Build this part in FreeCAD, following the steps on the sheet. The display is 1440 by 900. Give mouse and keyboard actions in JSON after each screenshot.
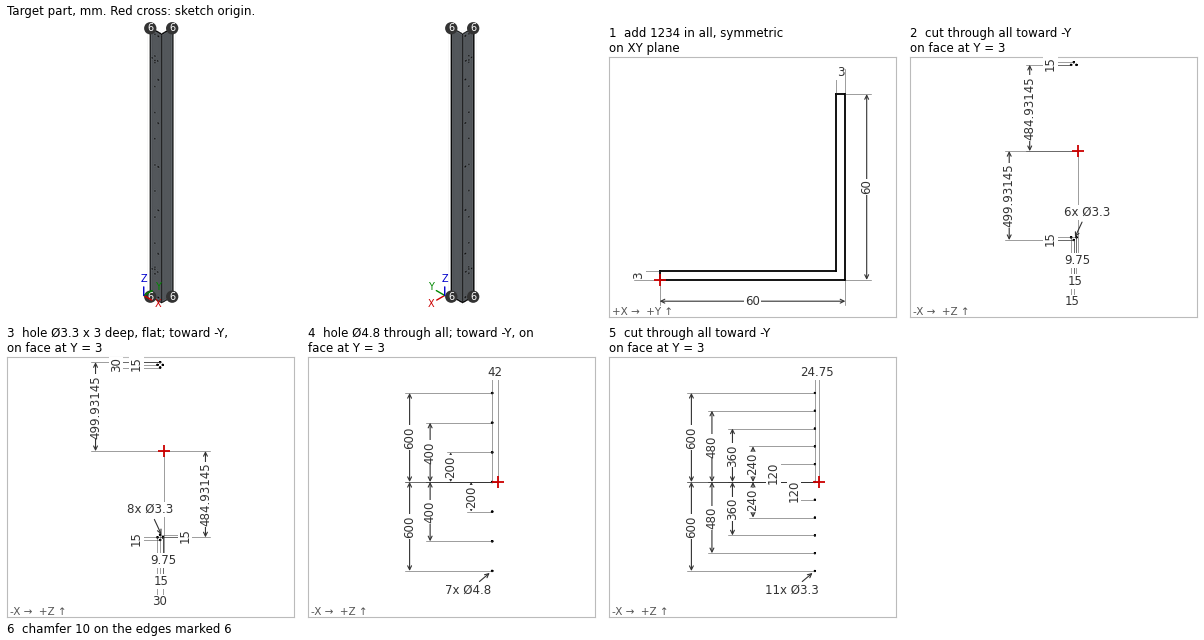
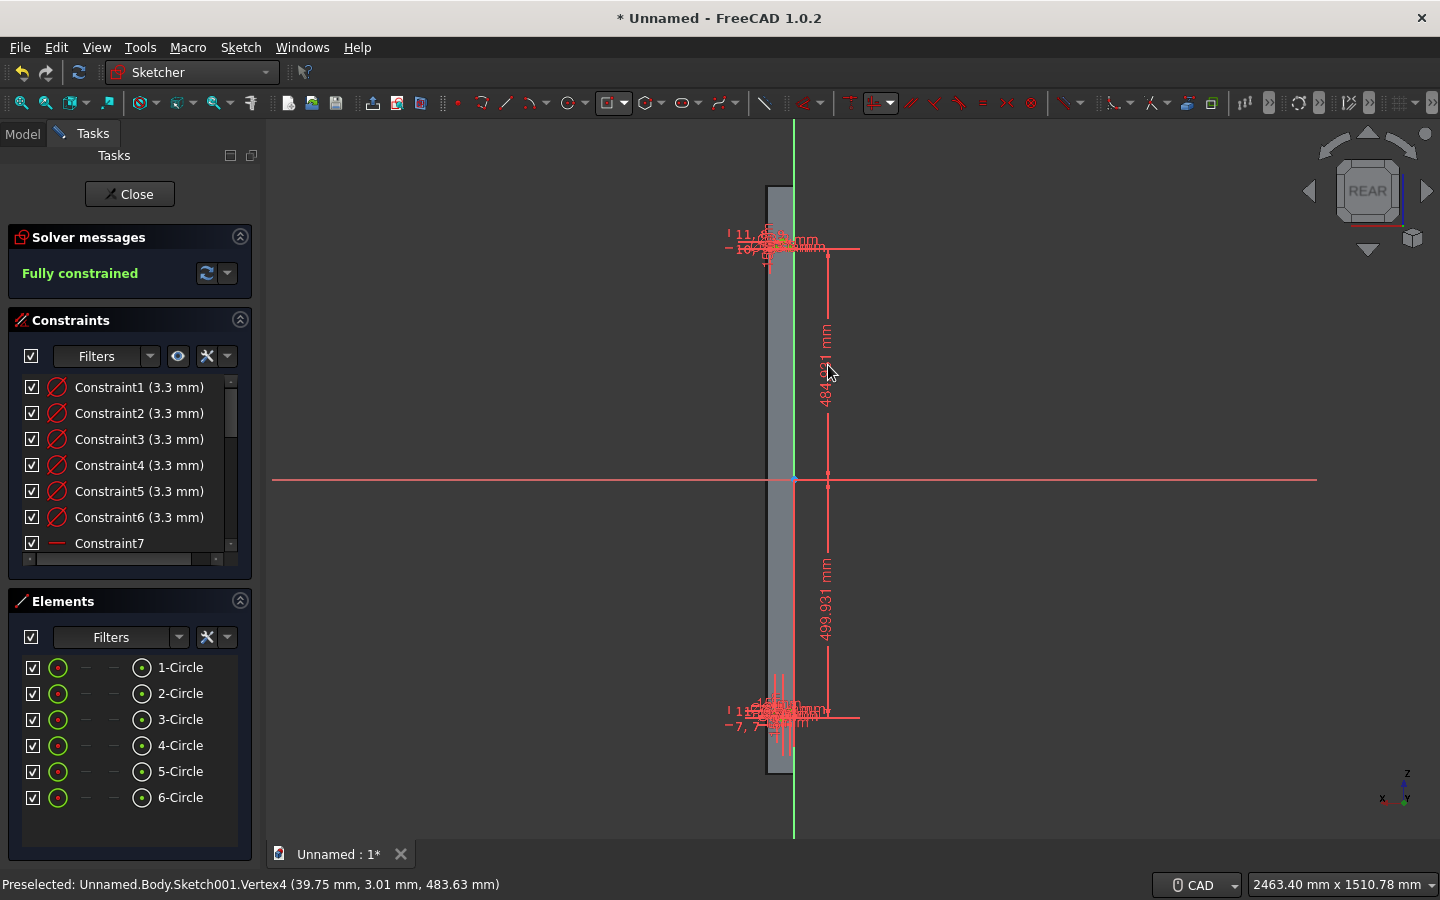
{"action": "left_click", "coordinate": [130, 194]}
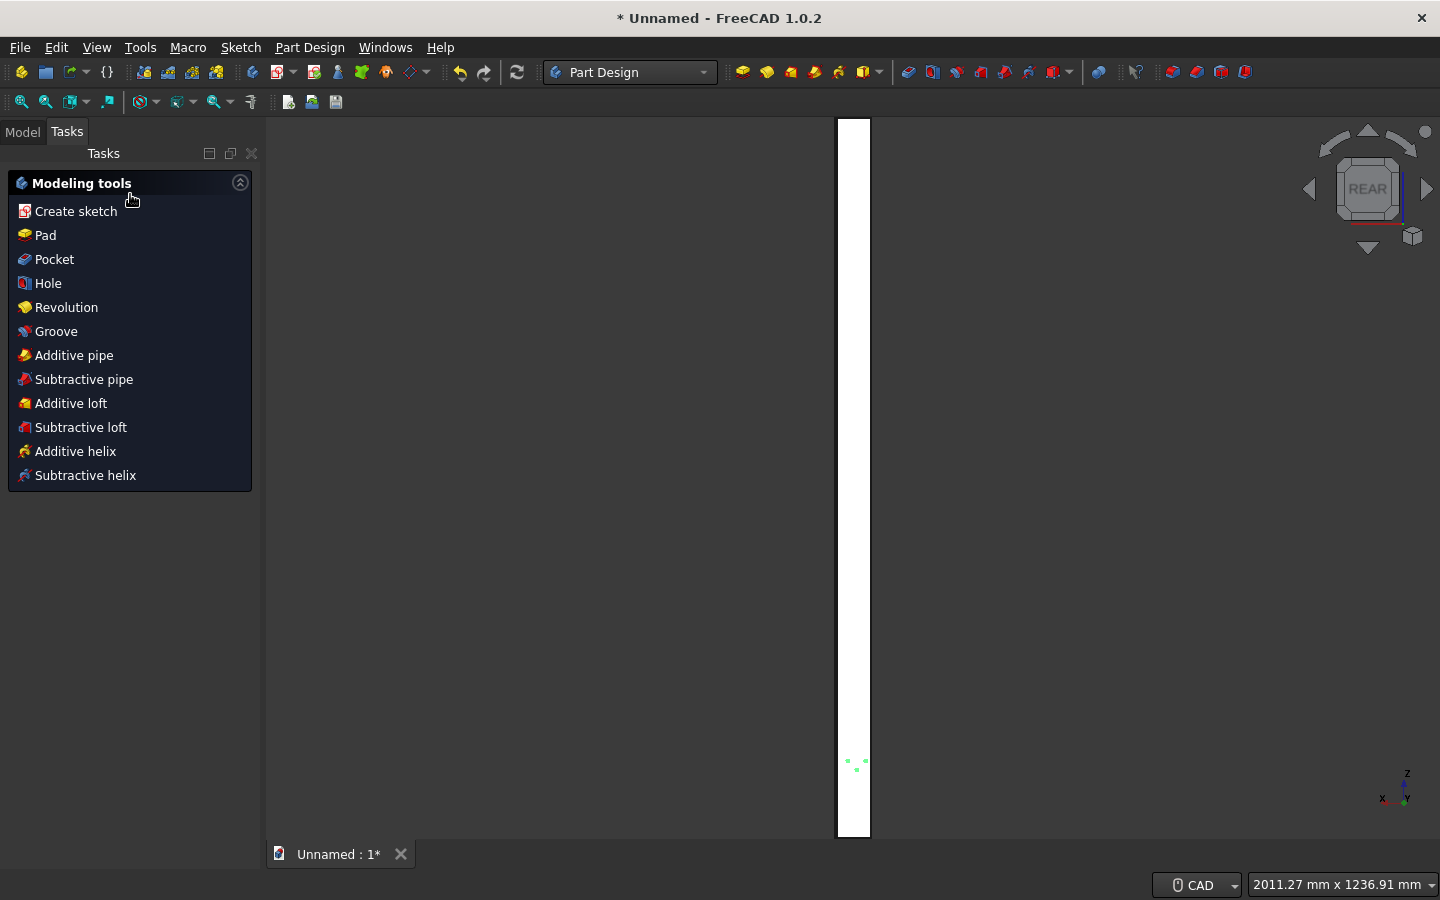
{"action": "left_click", "coordinate": [910, 72]}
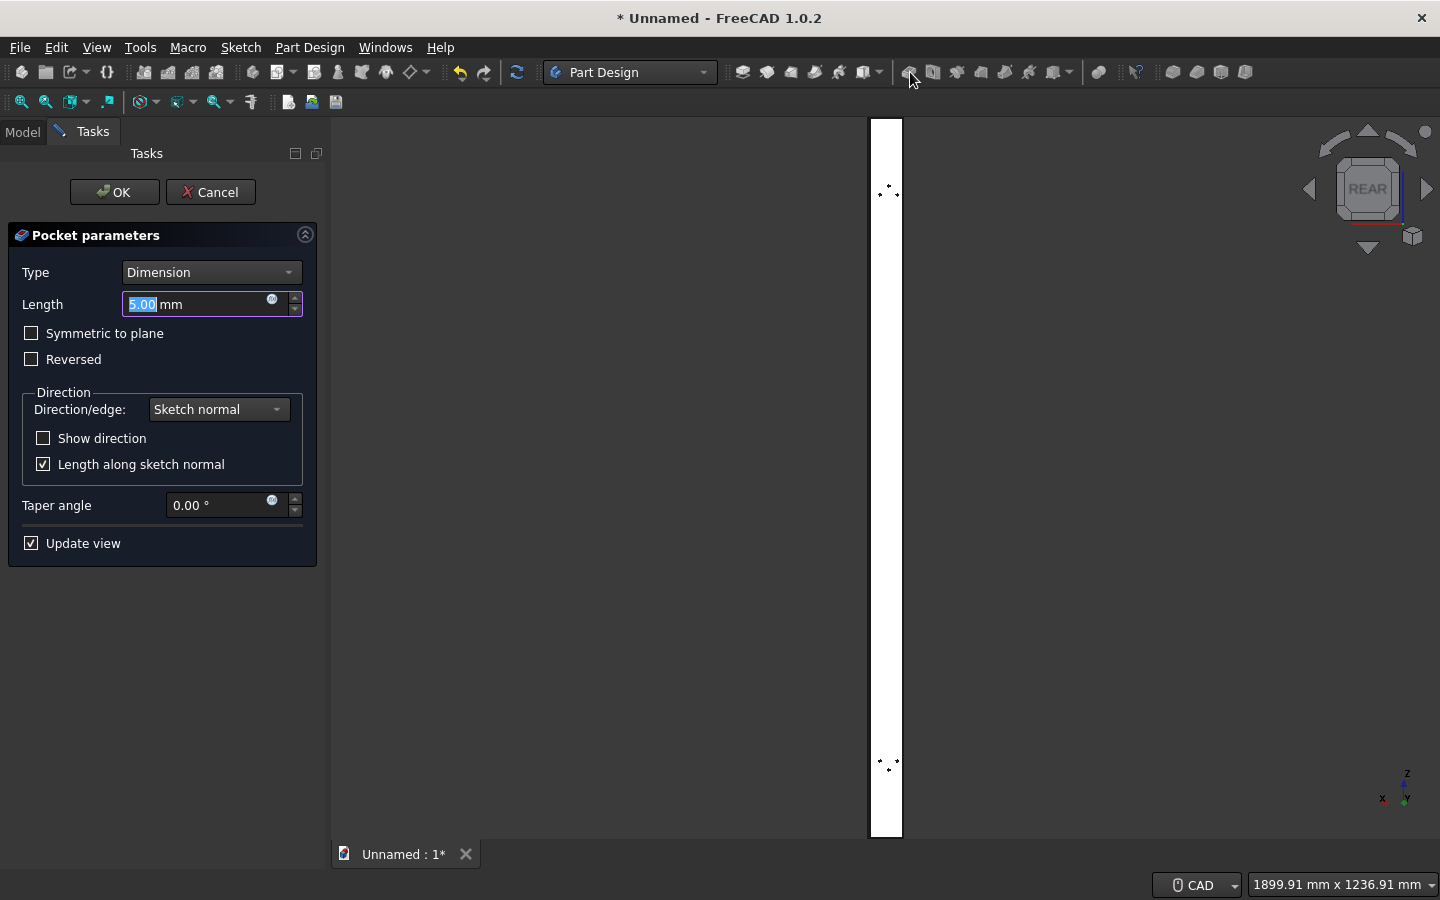
{"action": "left_click", "coordinate": [212, 272]}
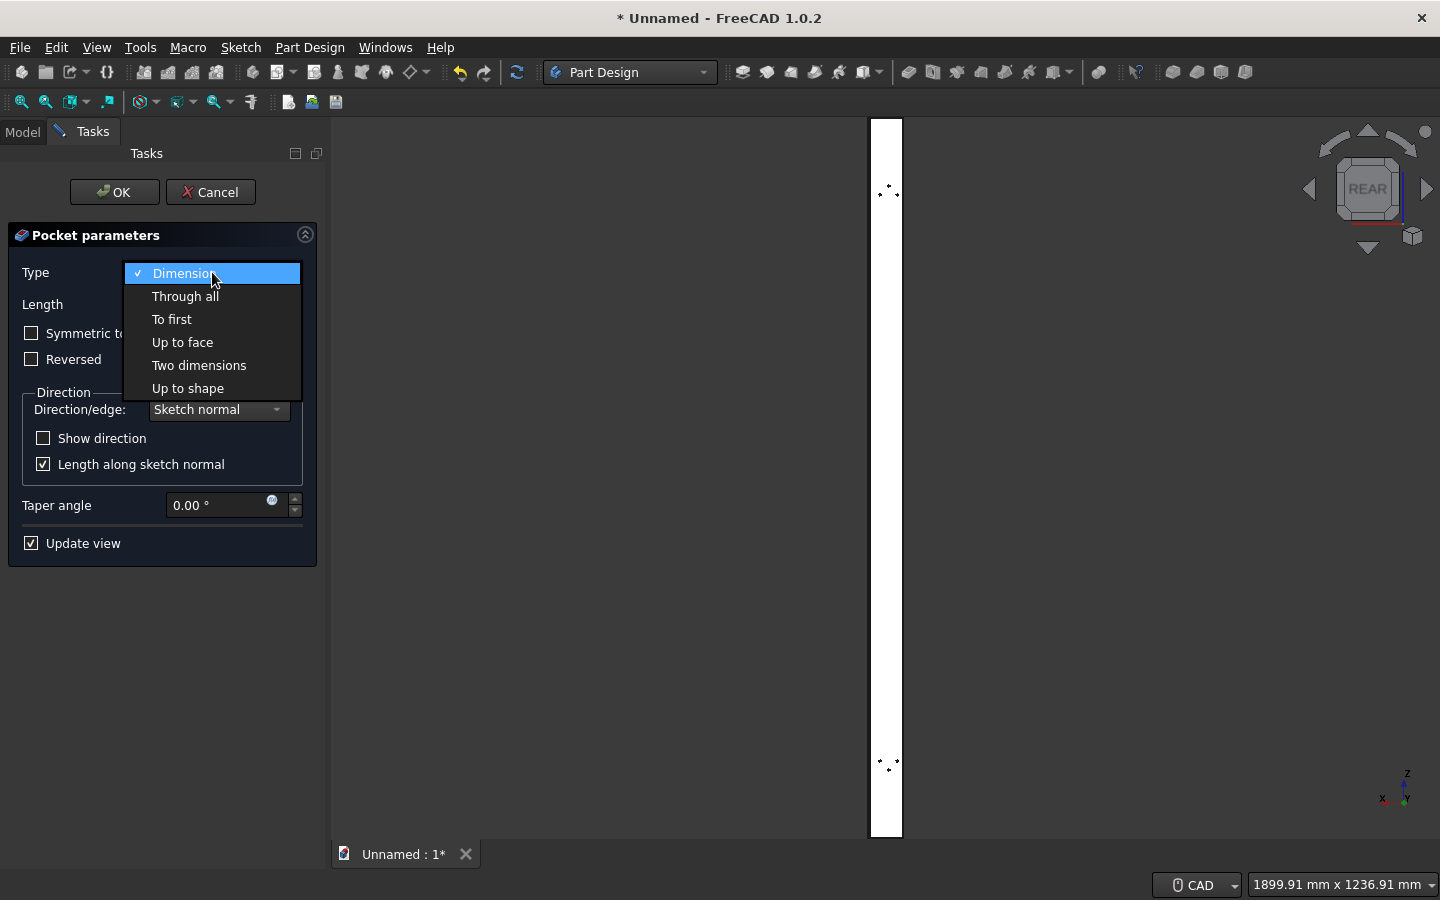
{"action": "left_click", "coordinate": [212, 296]}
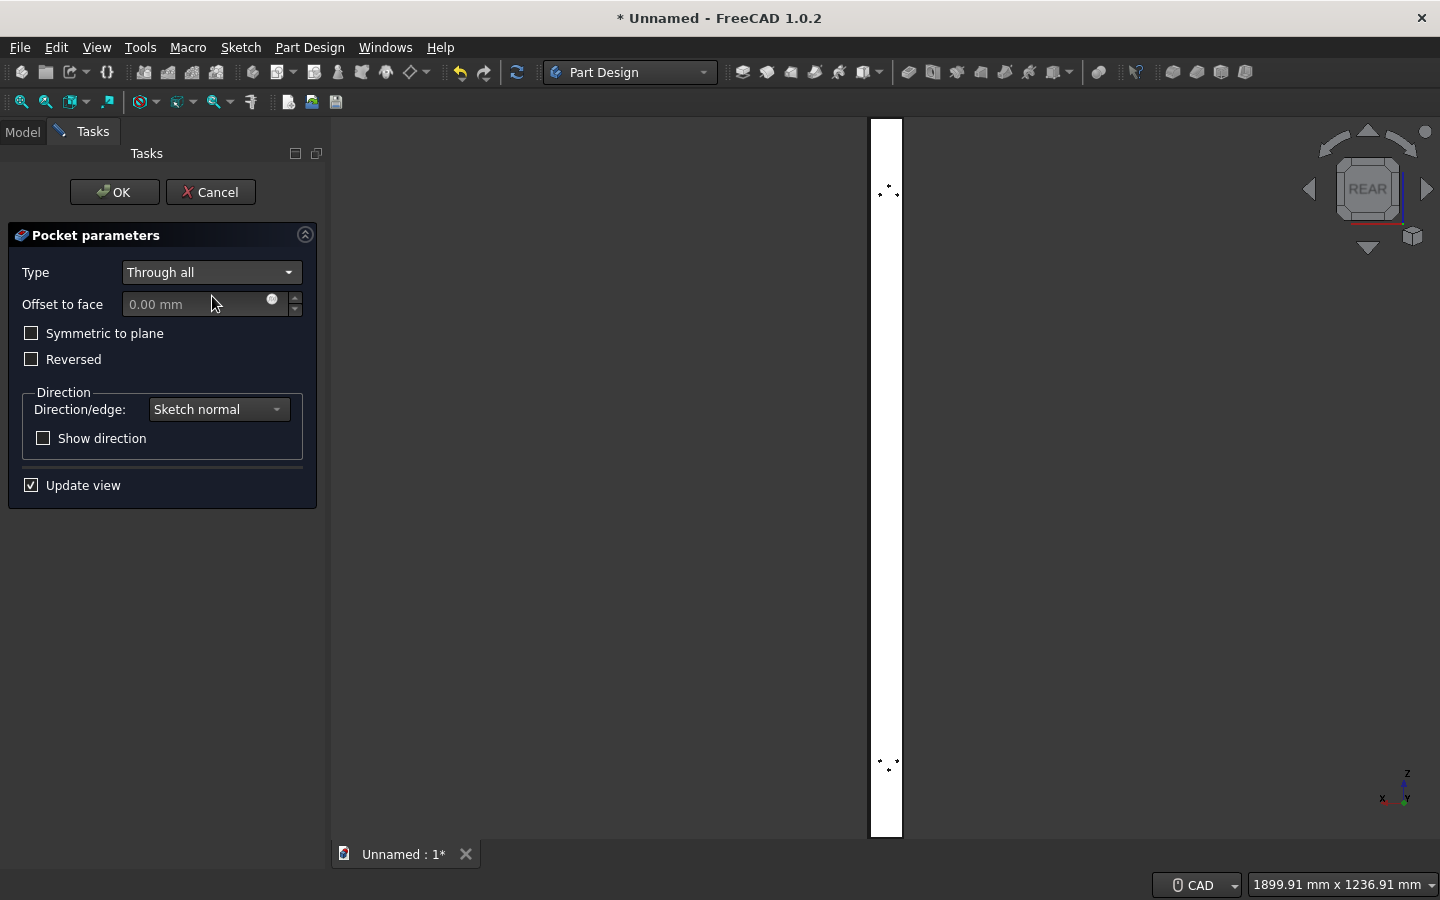
{"action": "left_click", "coordinate": [115, 192]}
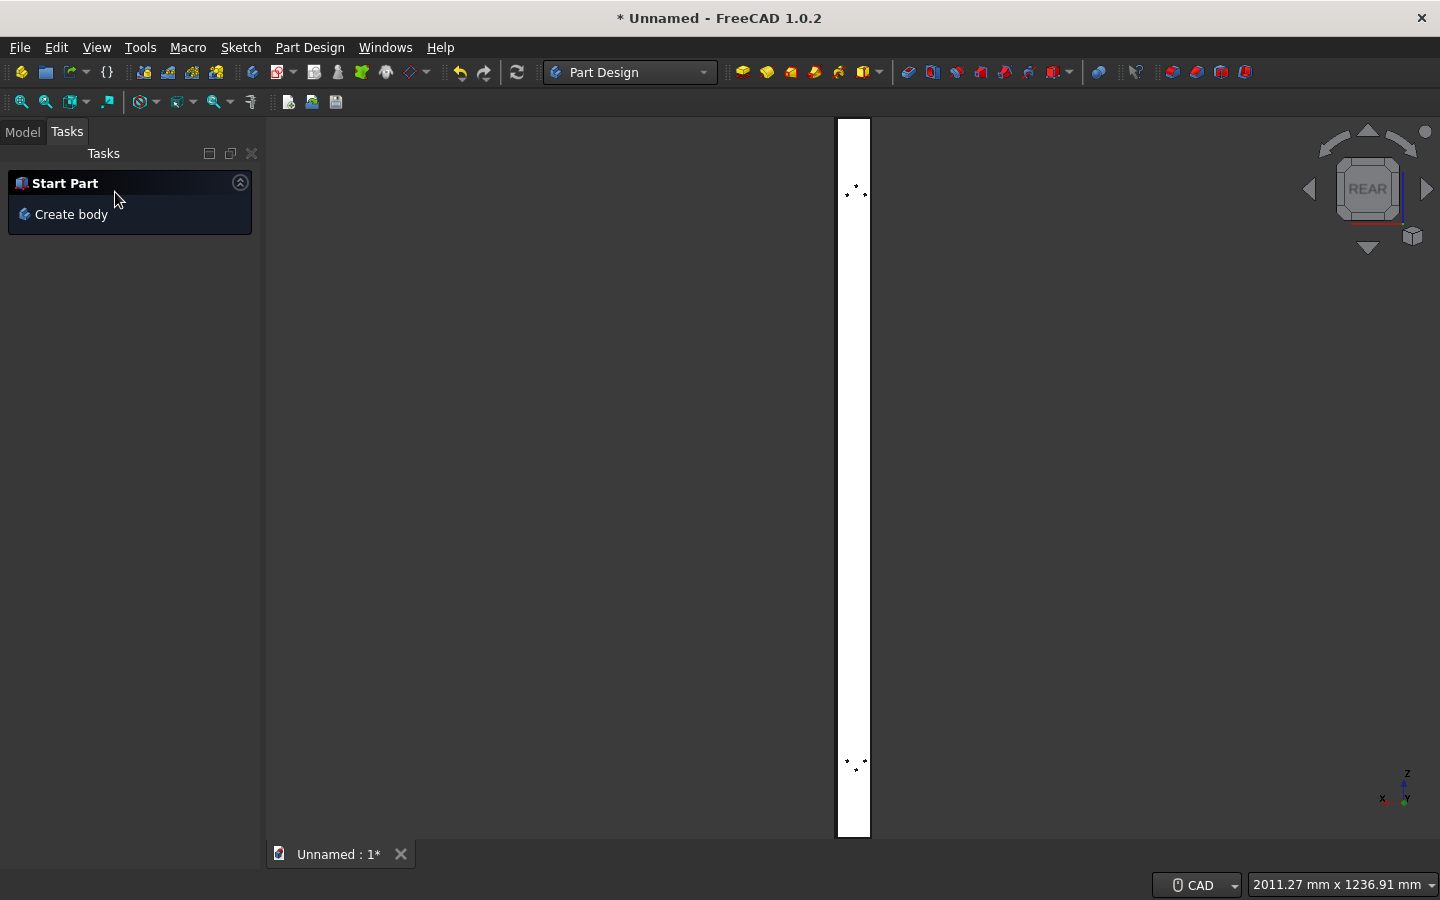
{"action": "left_click", "coordinate": [854, 271]}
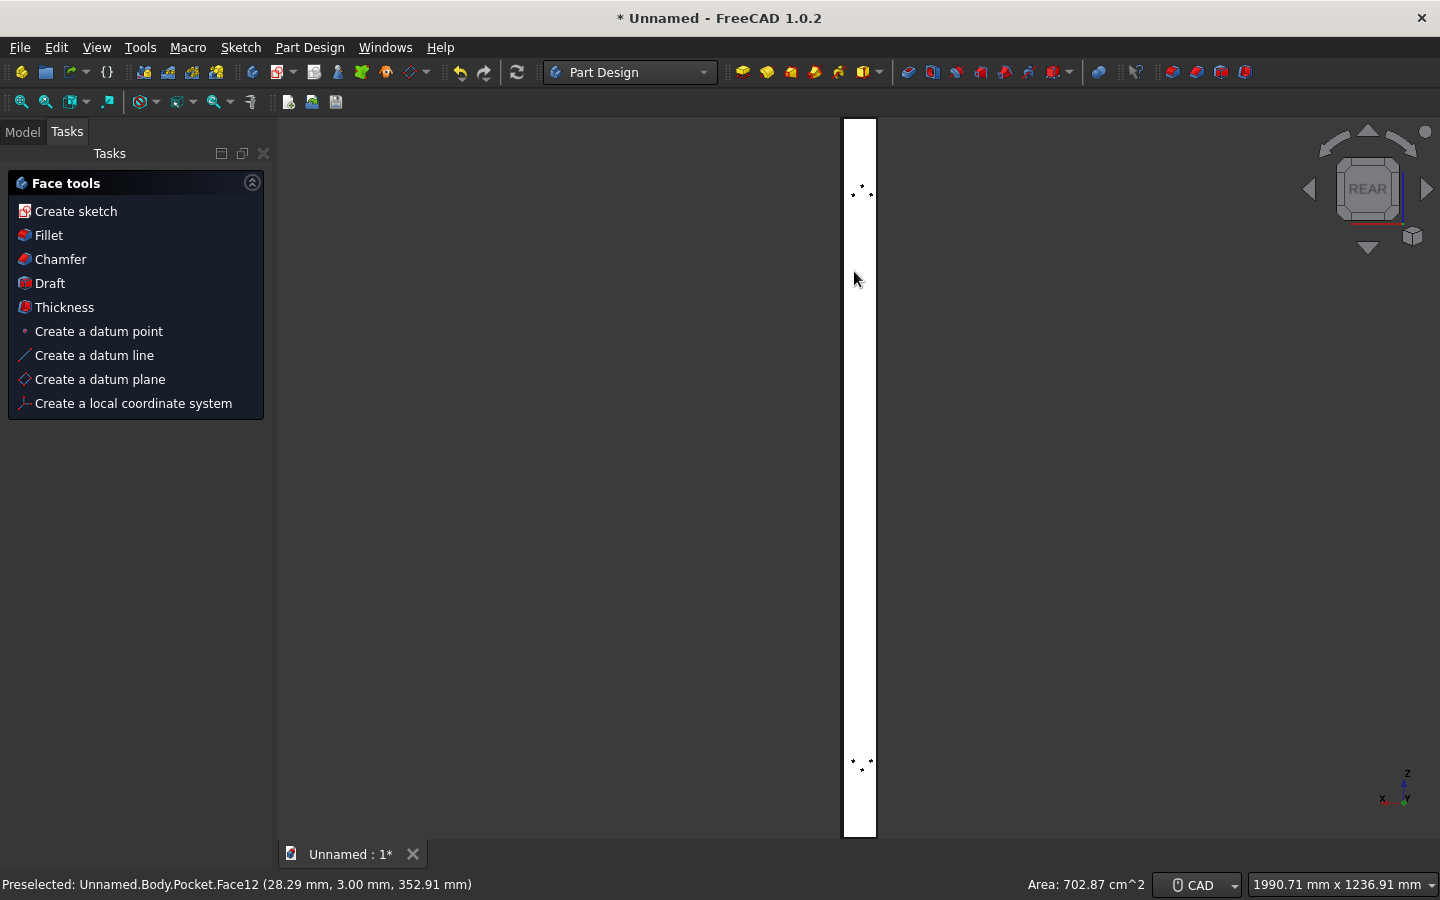
{"action": "left_click", "coordinate": [278, 72]}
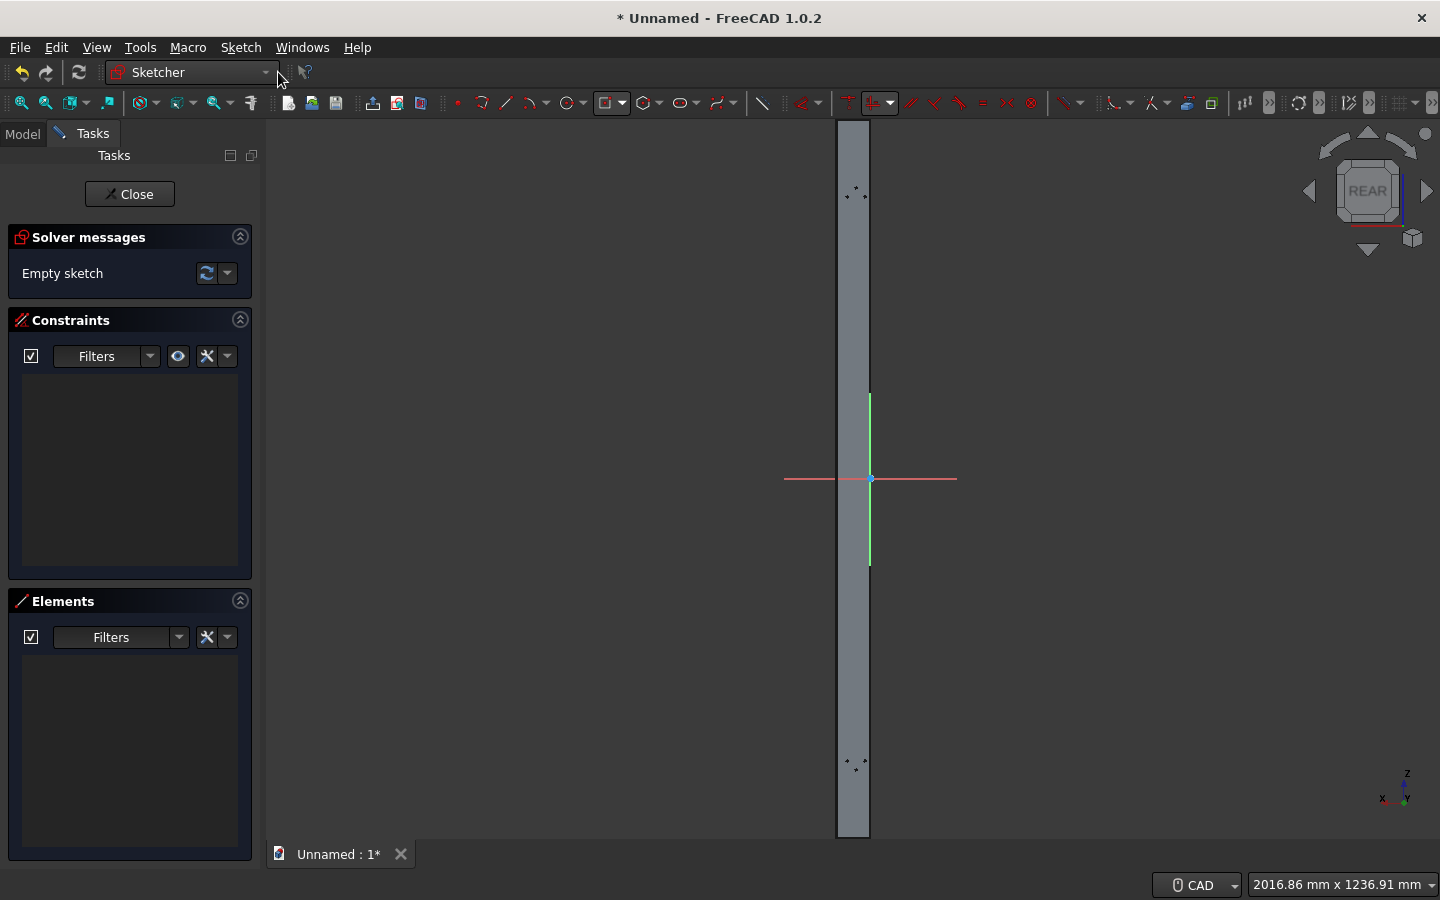
{"action": "left_click", "coordinate": [422, 104]}